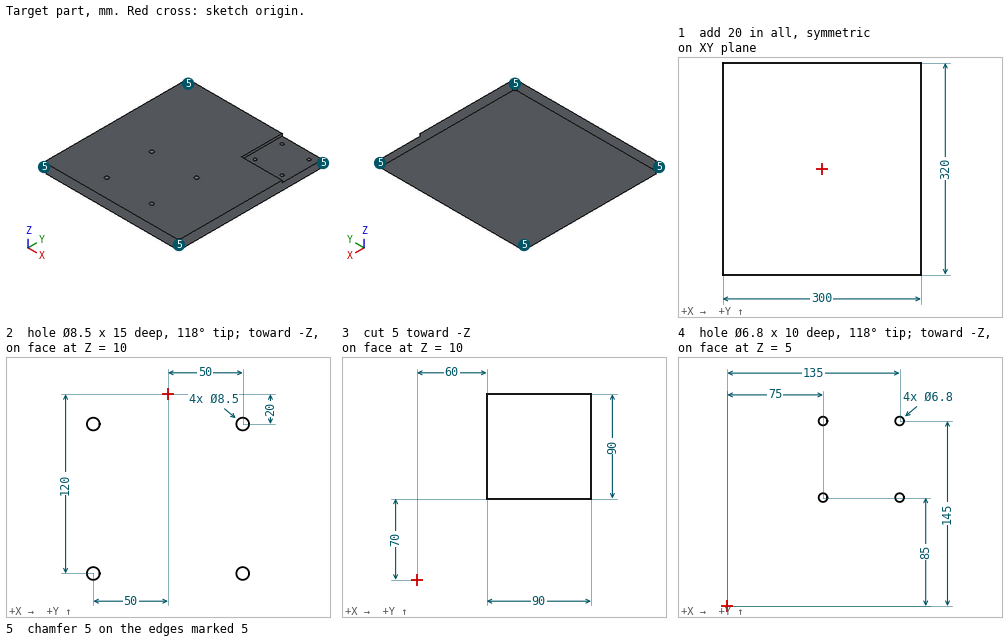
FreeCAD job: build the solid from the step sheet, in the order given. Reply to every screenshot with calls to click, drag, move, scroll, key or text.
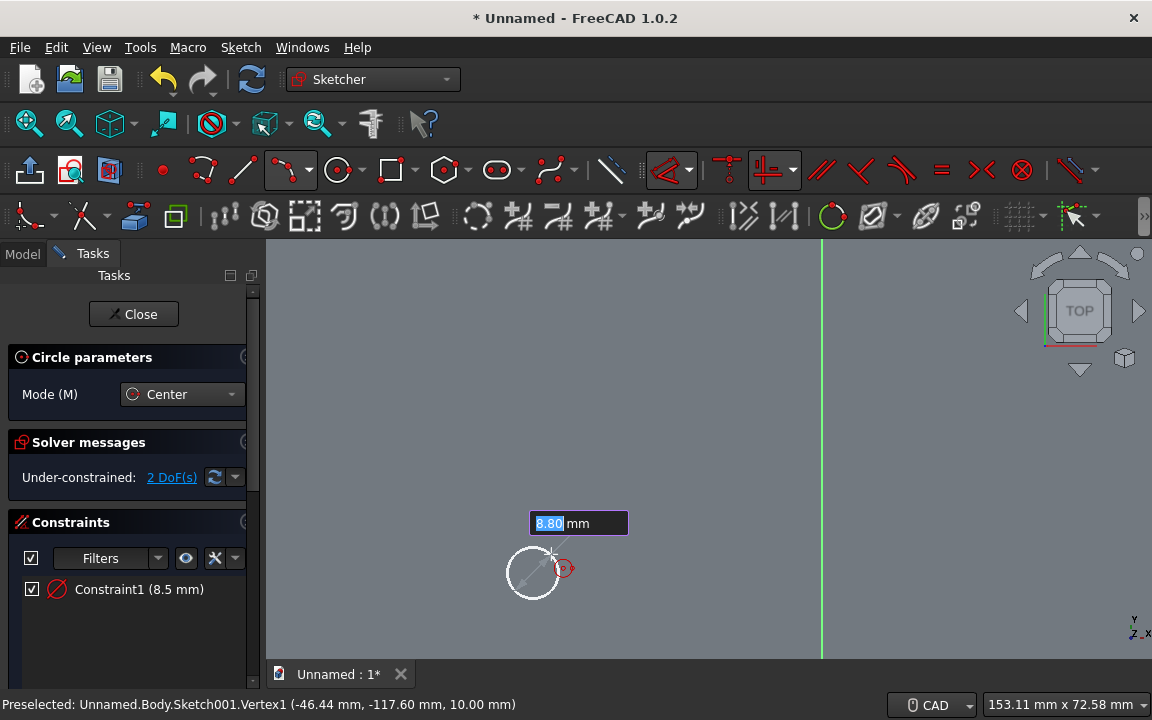
text(8.5)
key(Return)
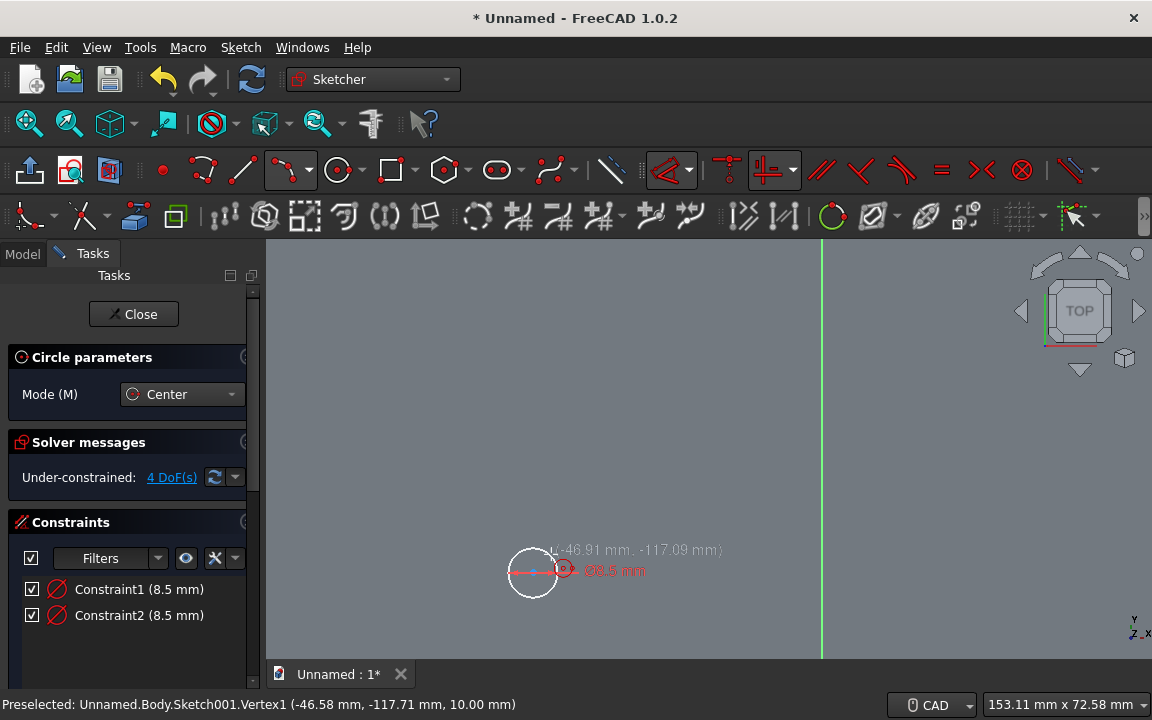
scroll(535, 572, down, 5)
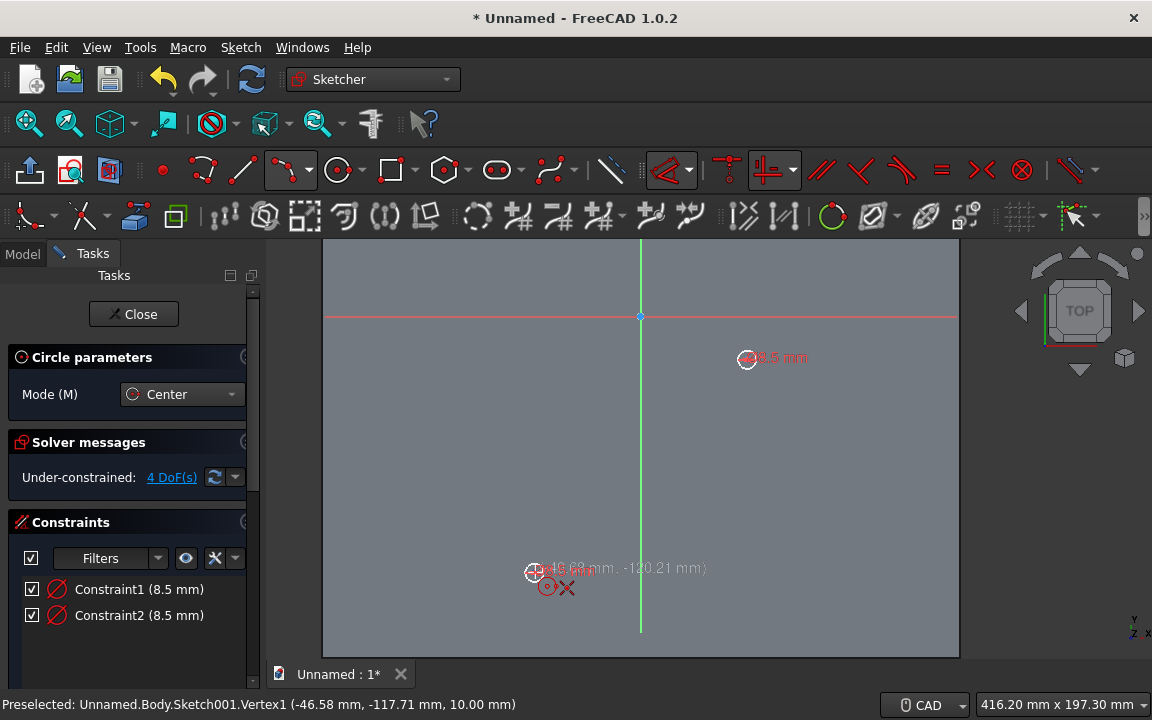
scroll(535, 360, up, 5)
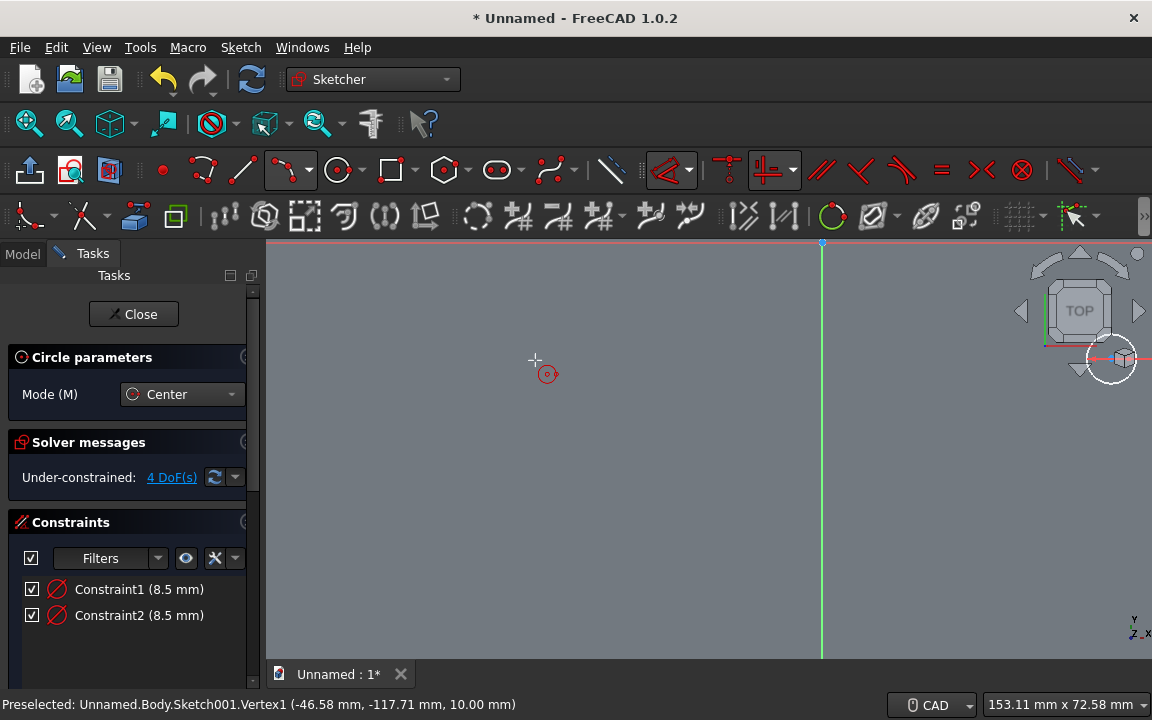
click(533, 358)
move(551, 341)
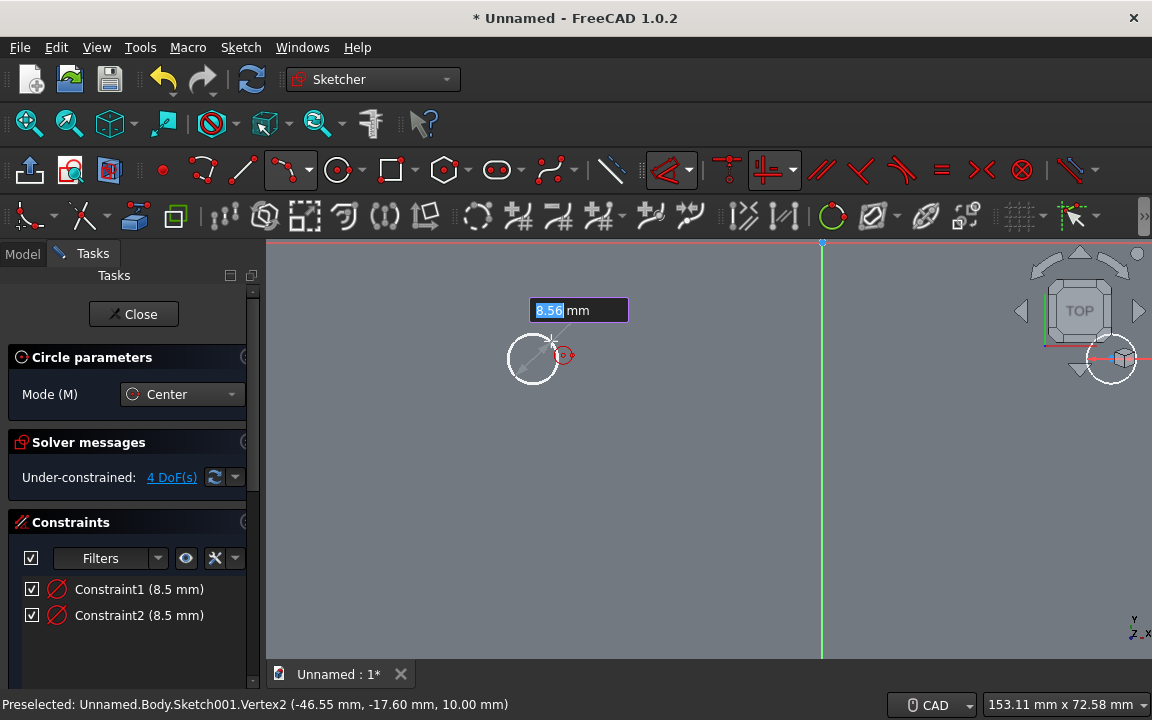
text(8.5)
key(Return)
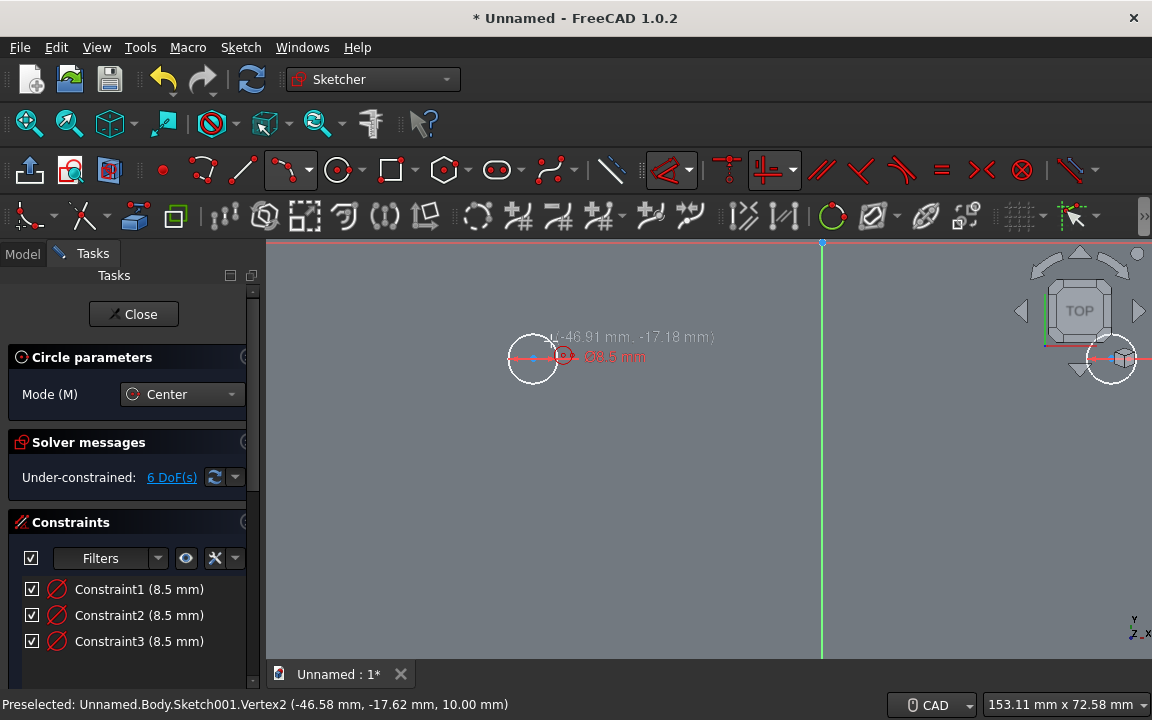
scroll(535, 360, down, 5)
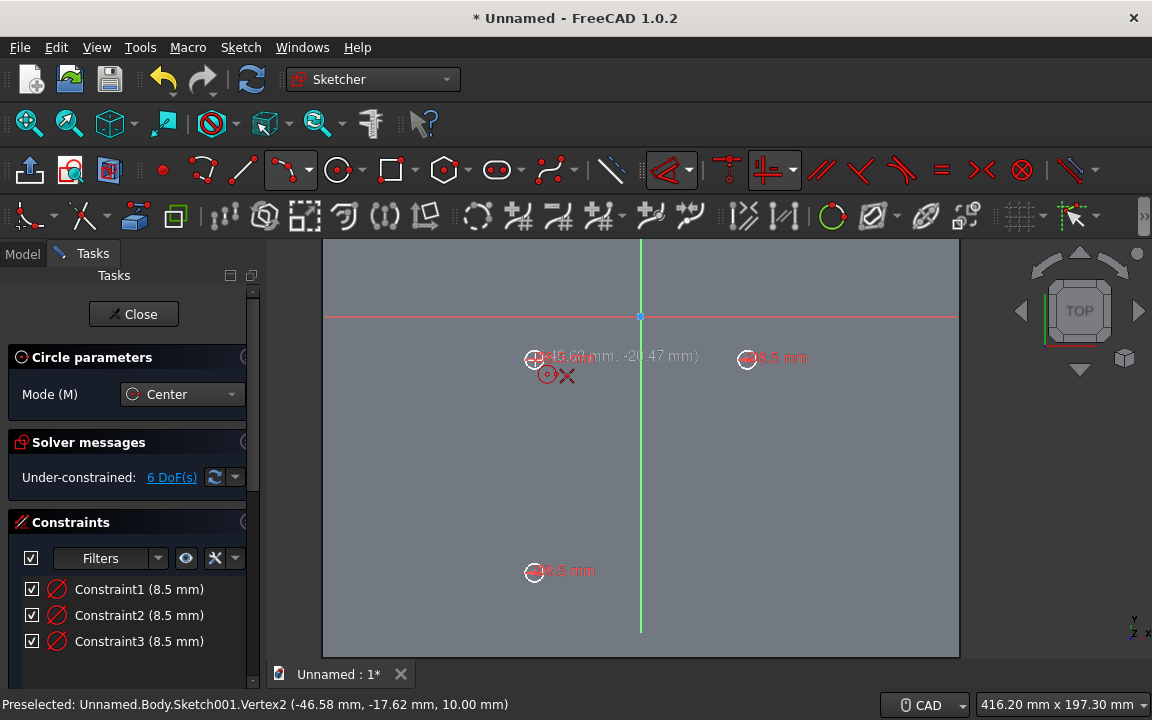
scroll(747, 572, up, 5)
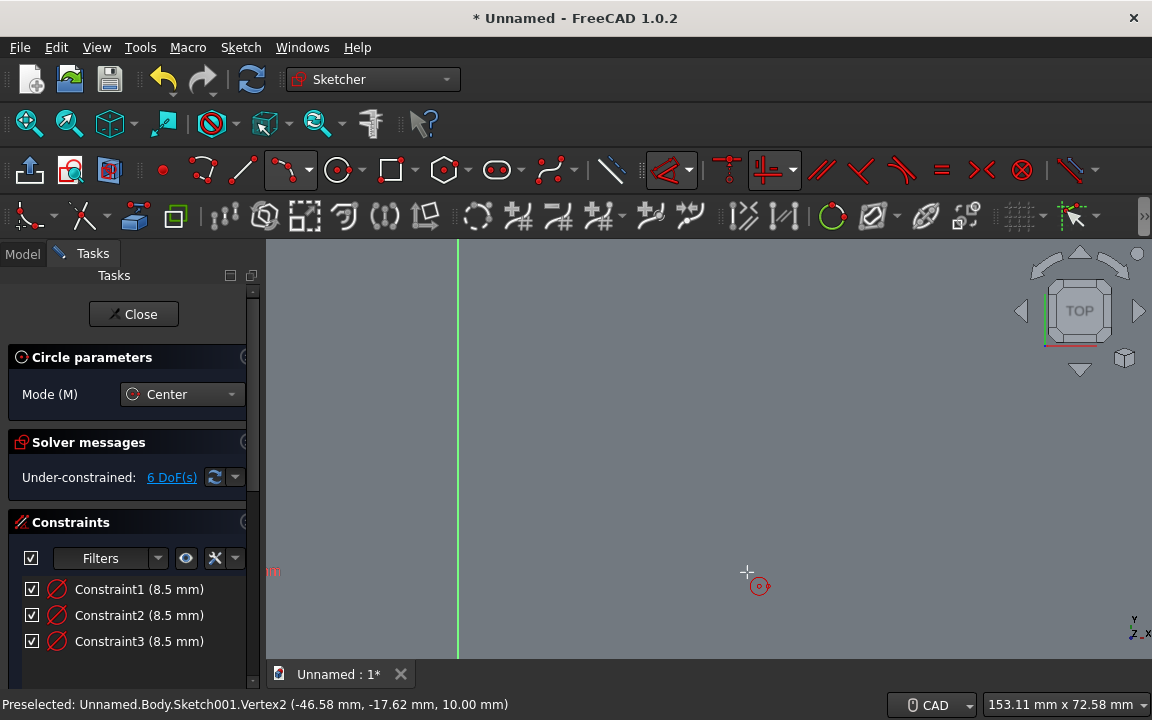
click(747, 572)
move(764, 554)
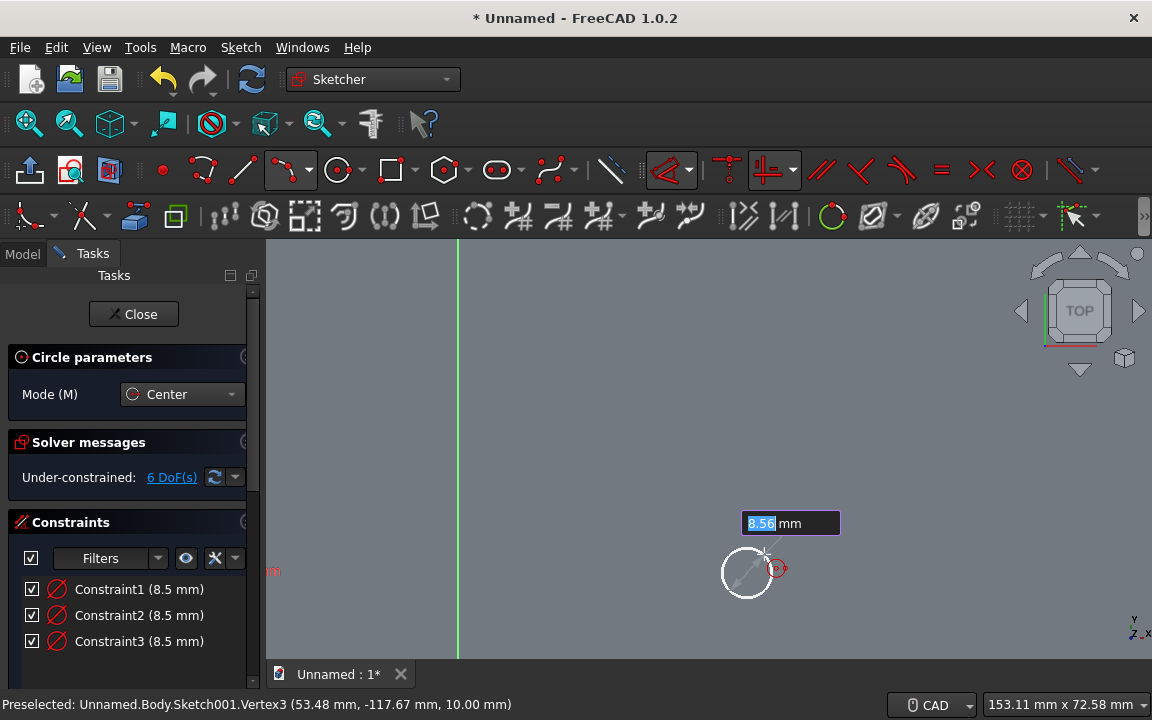
text(8.5)
key(Return)
key(Escape)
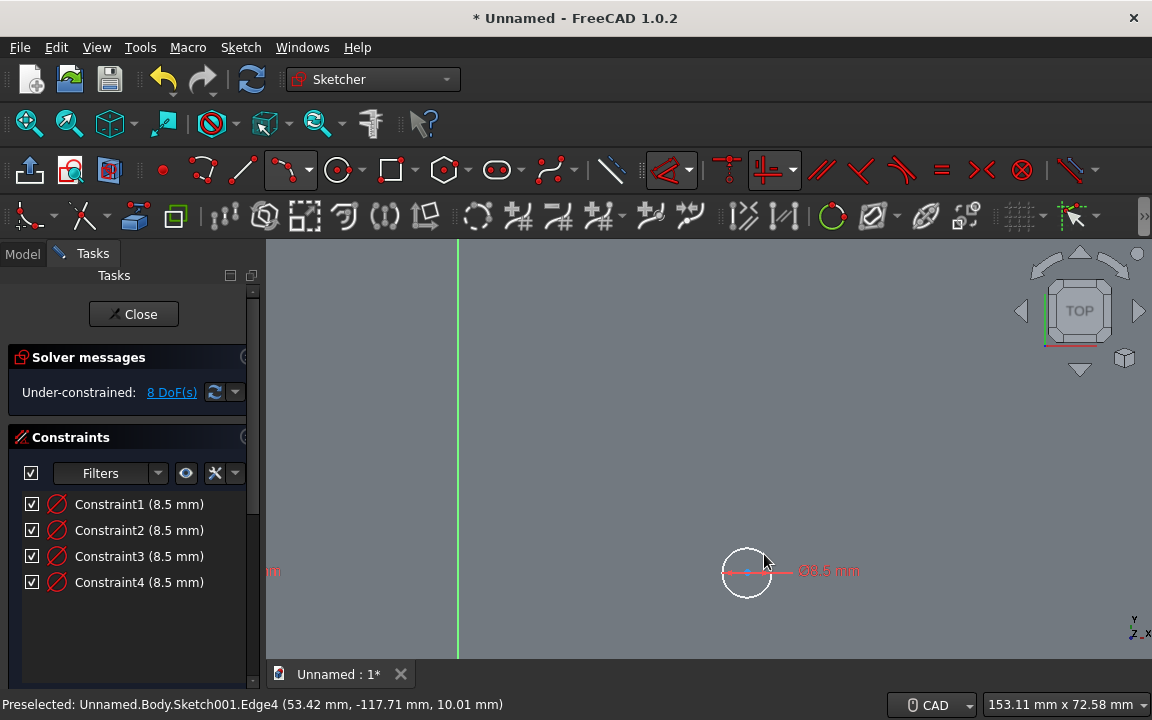
scroll(747, 572, down, 5)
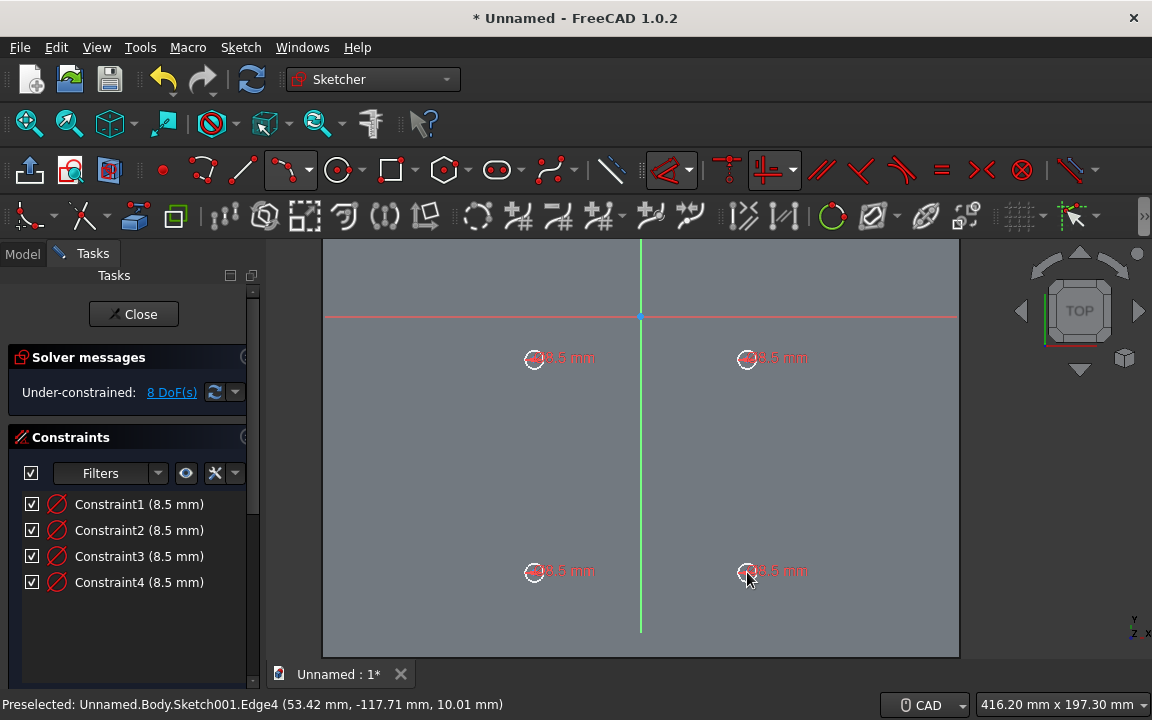
click(534, 573)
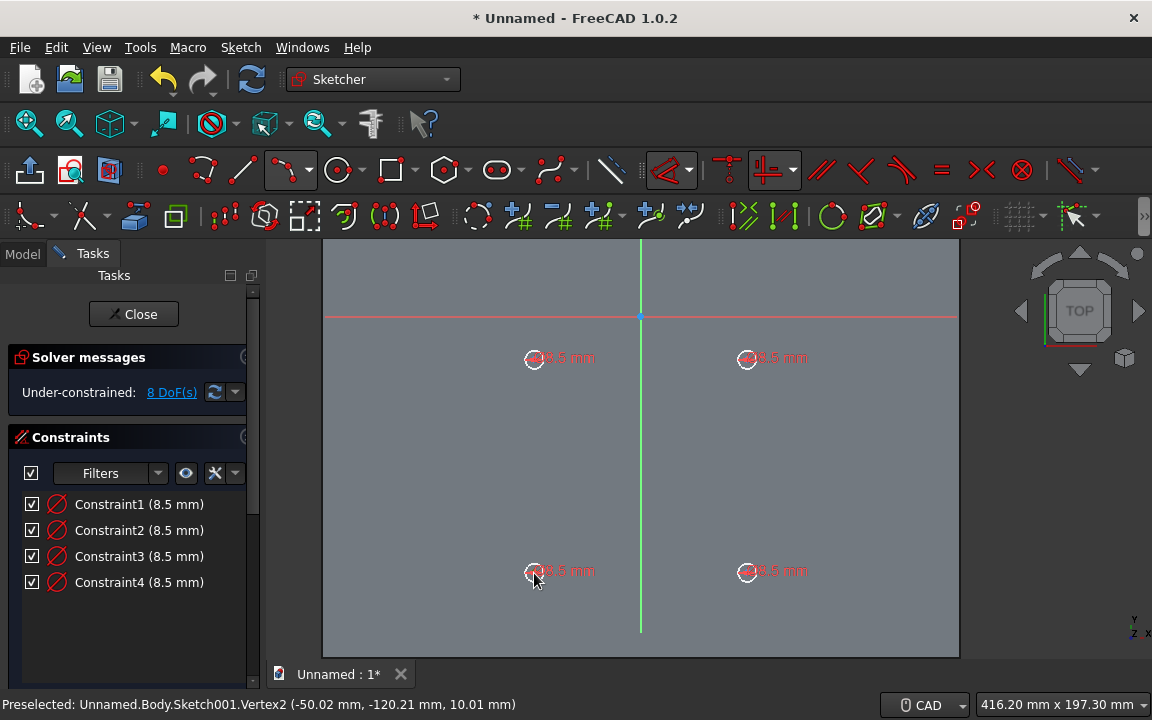
click(534, 360)